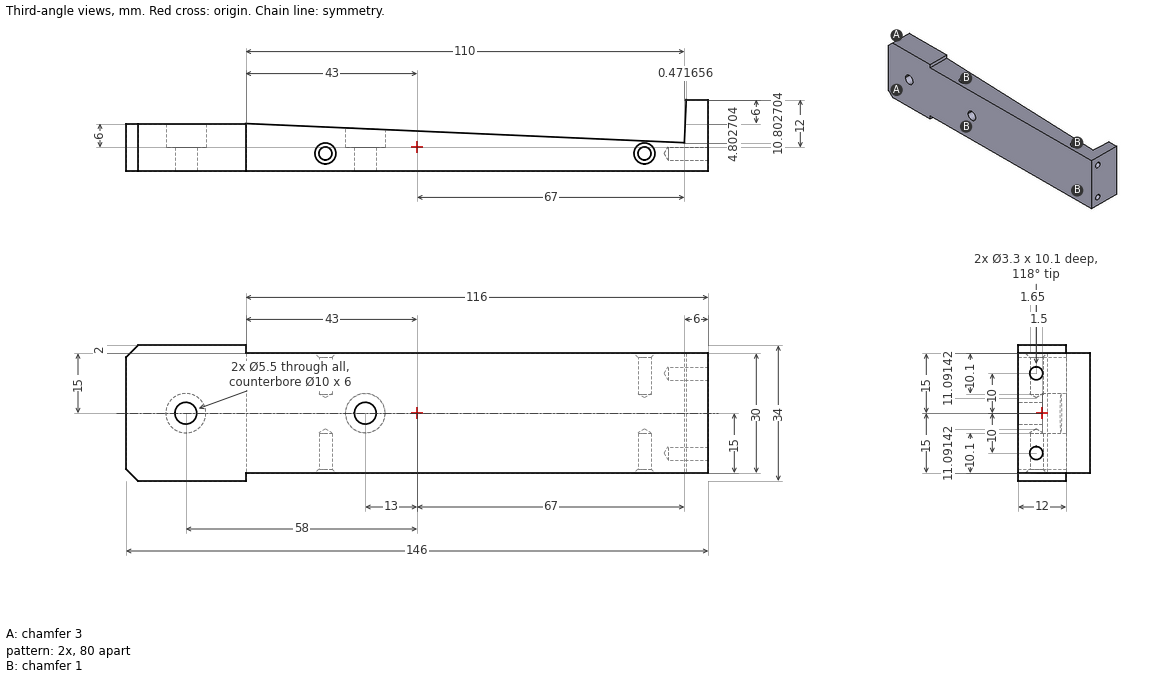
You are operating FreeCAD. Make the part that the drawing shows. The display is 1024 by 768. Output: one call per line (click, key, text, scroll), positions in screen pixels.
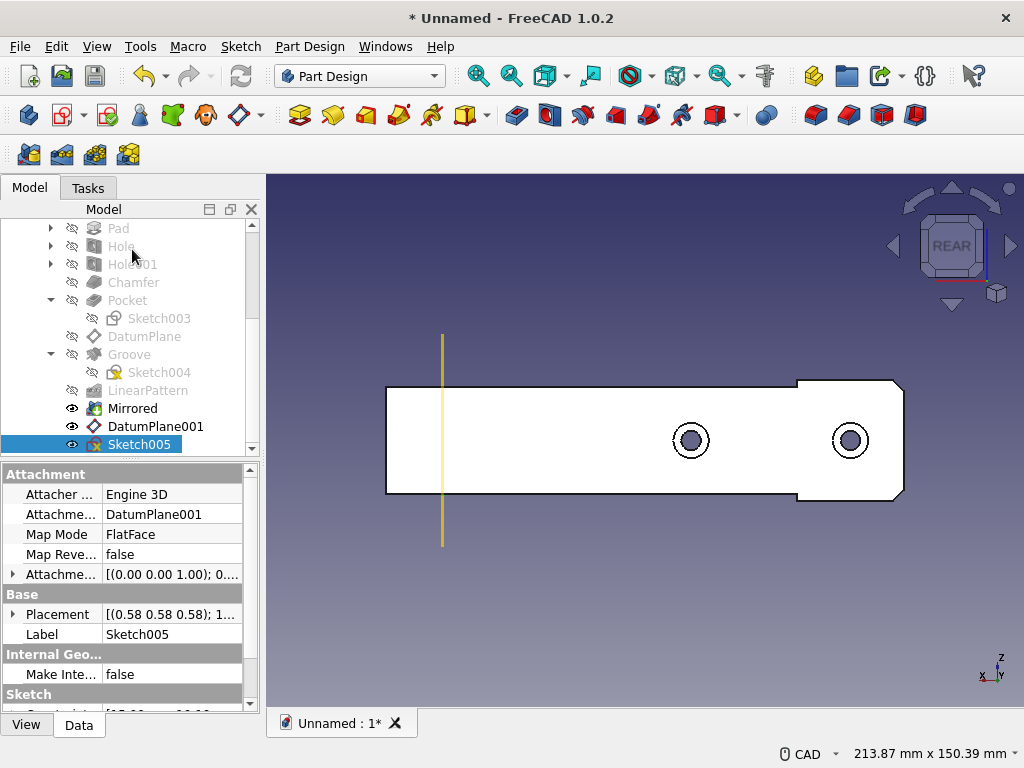
click(583, 116)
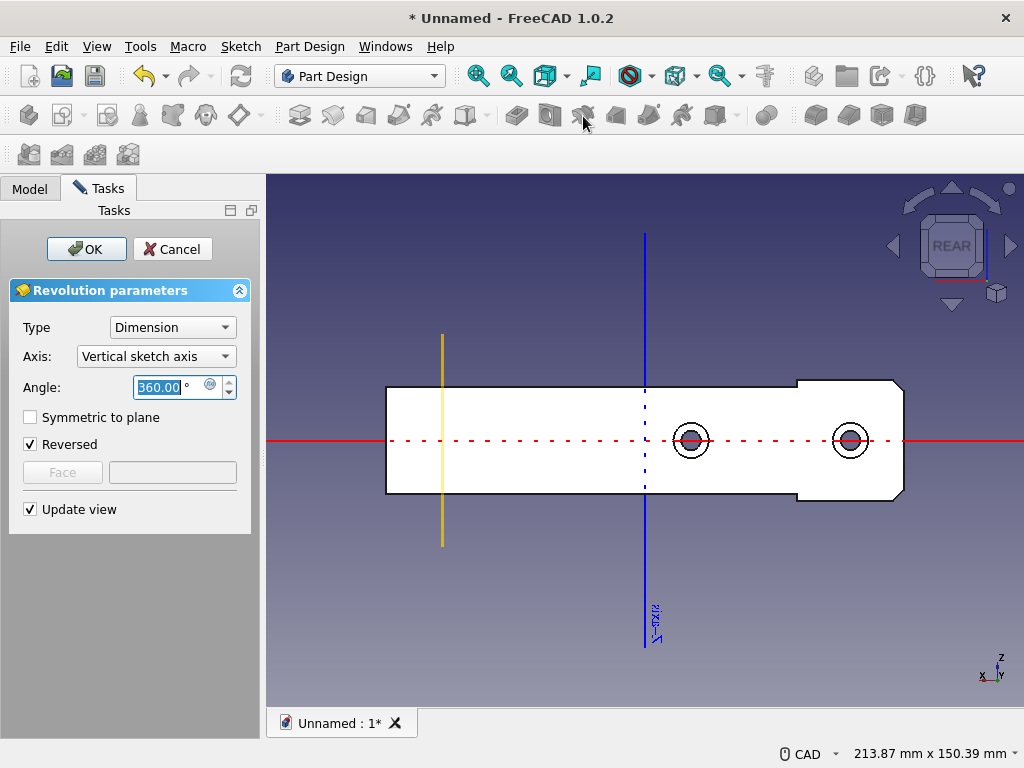
click(157, 356)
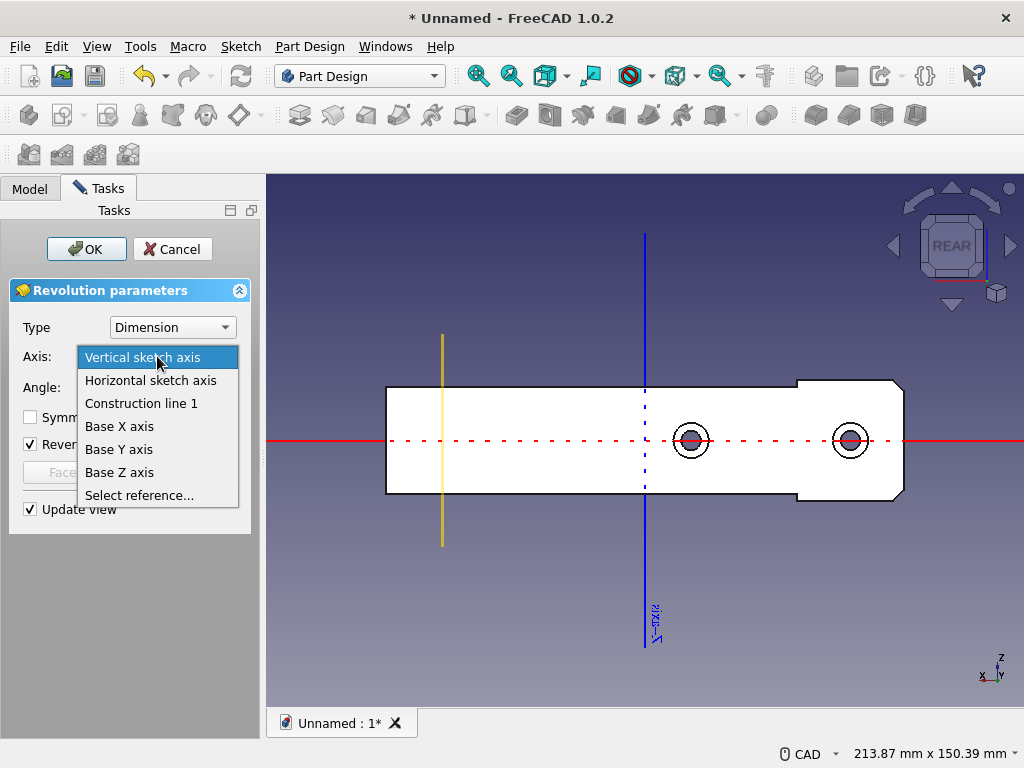
click(156, 404)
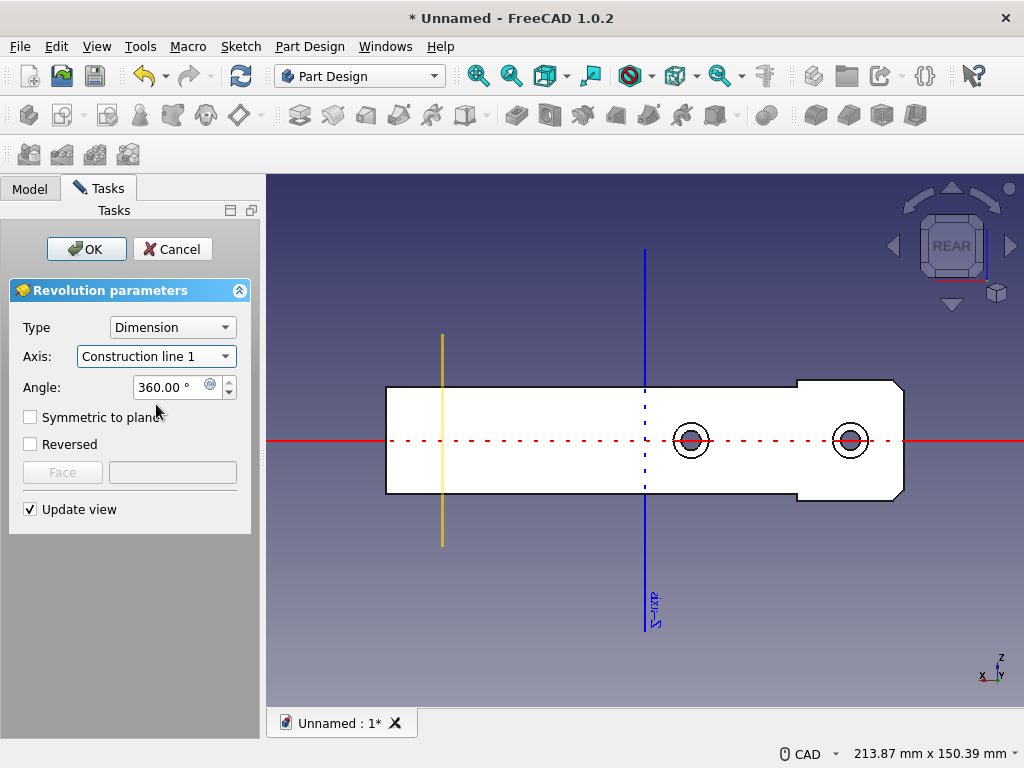
click(87, 249)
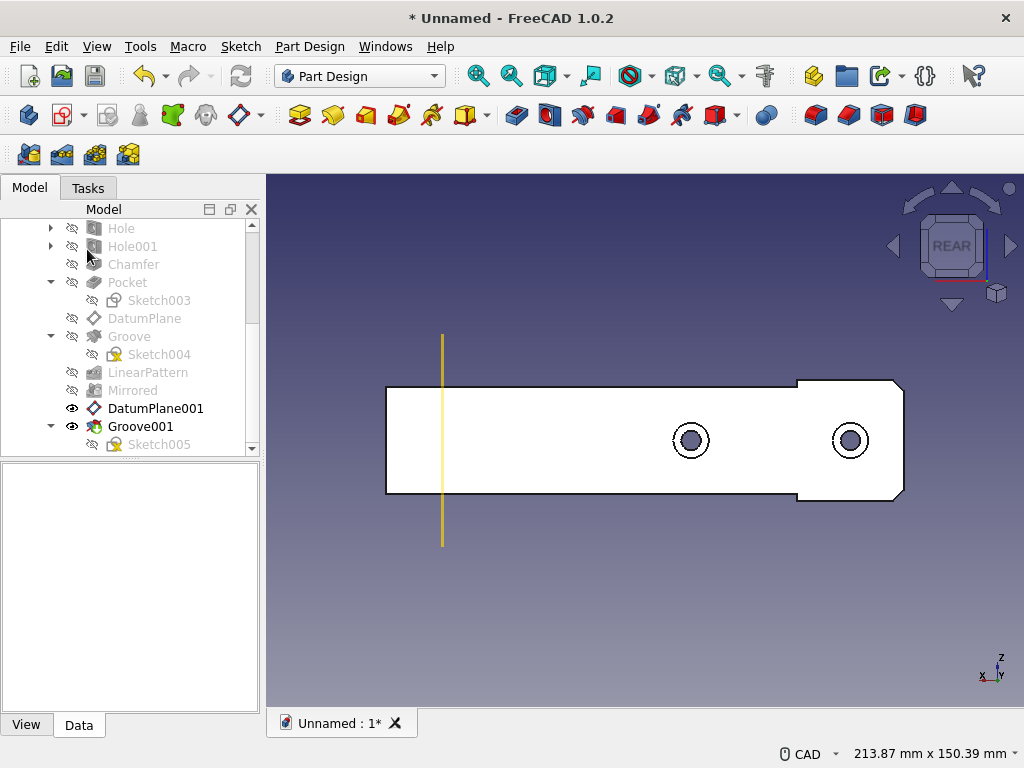
click(117, 408)
key(space)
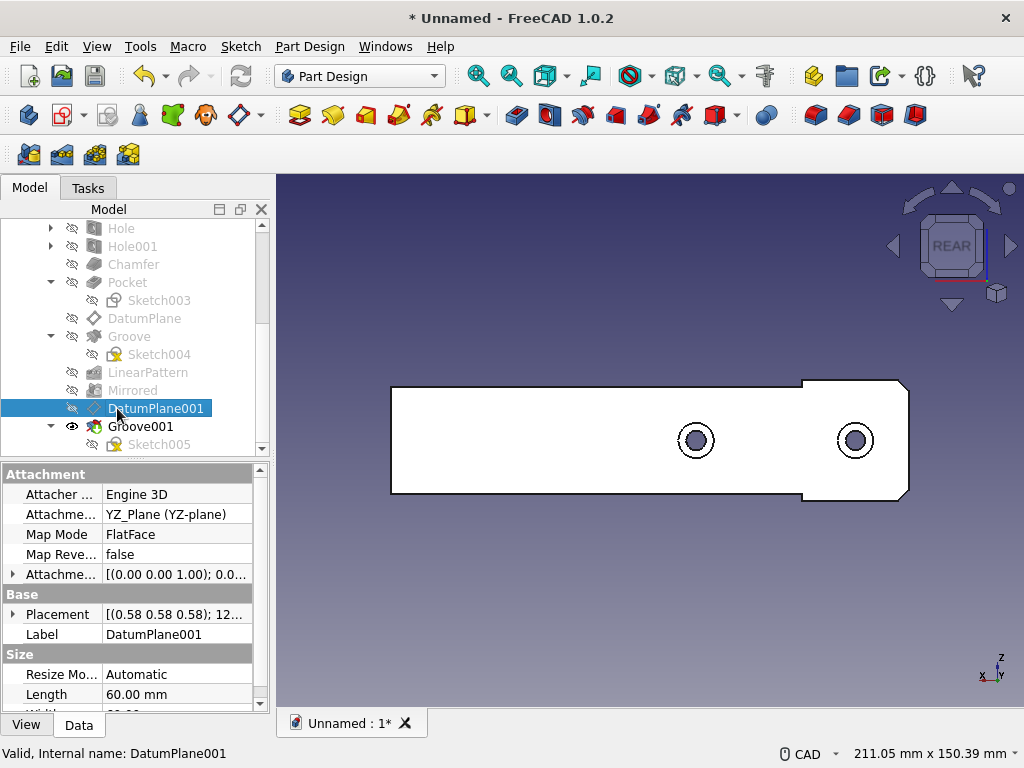
click(502, 439)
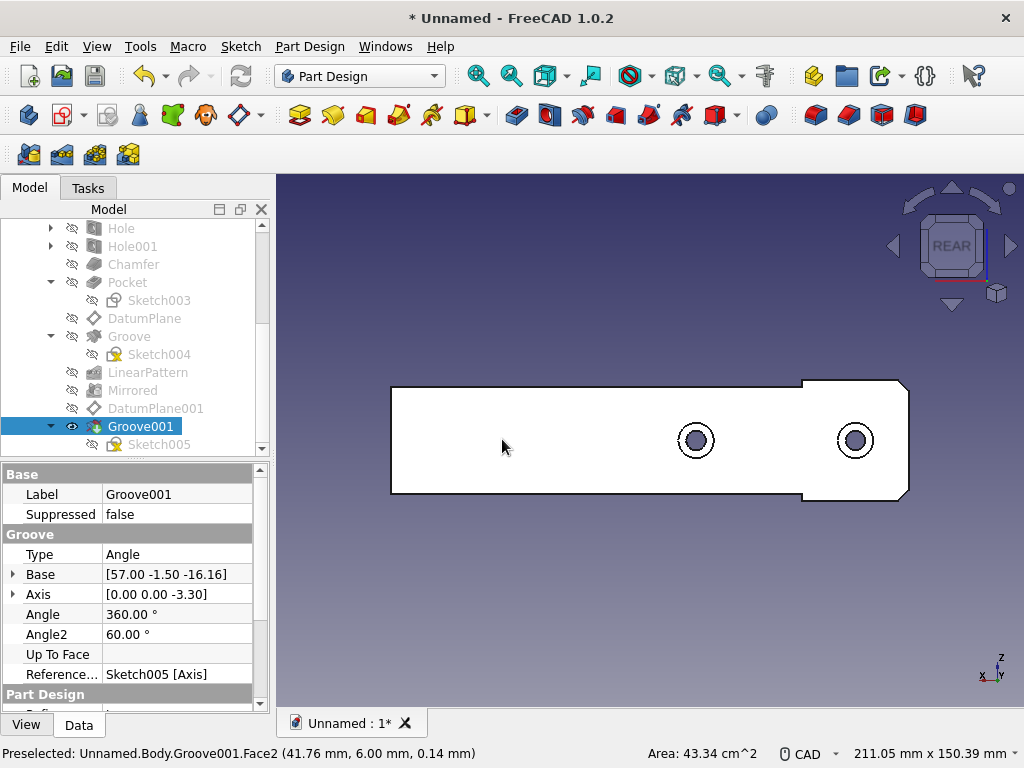
click(62, 116)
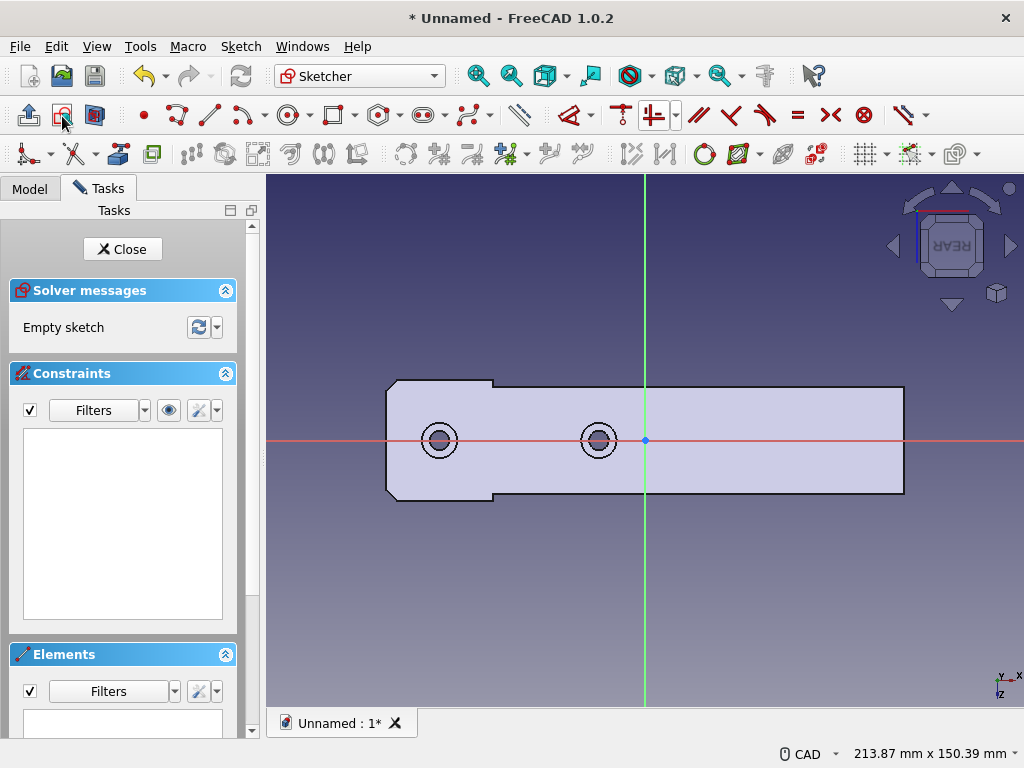
scroll(294, 441, down, 1)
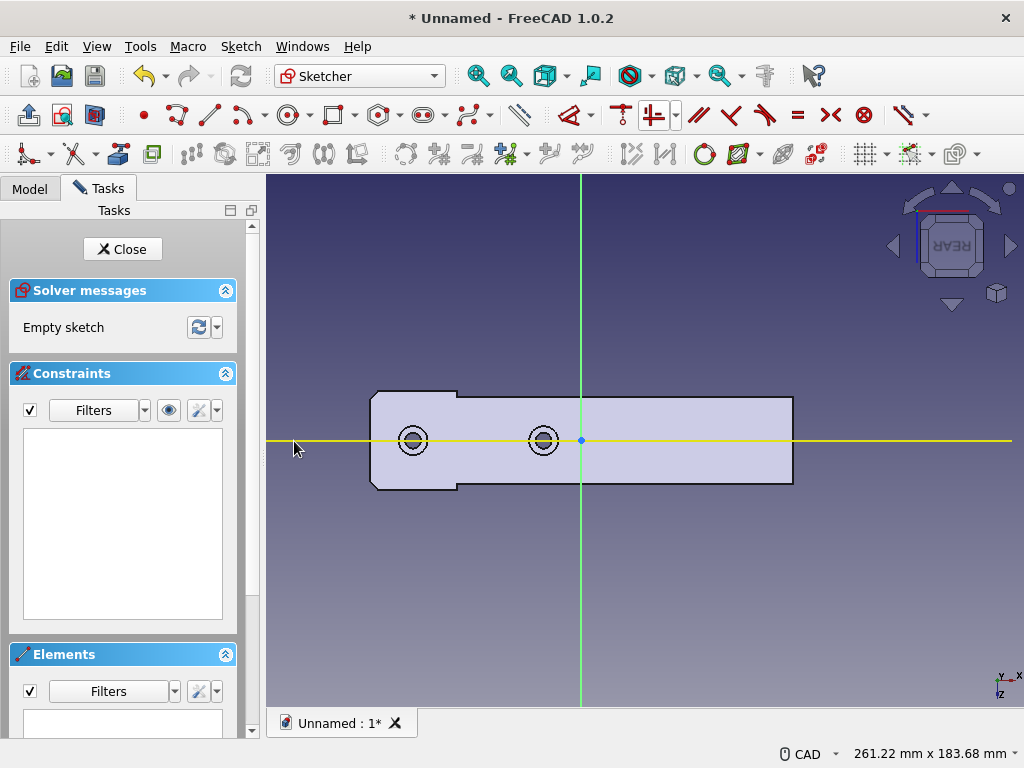
scroll(822, 441, up, 3)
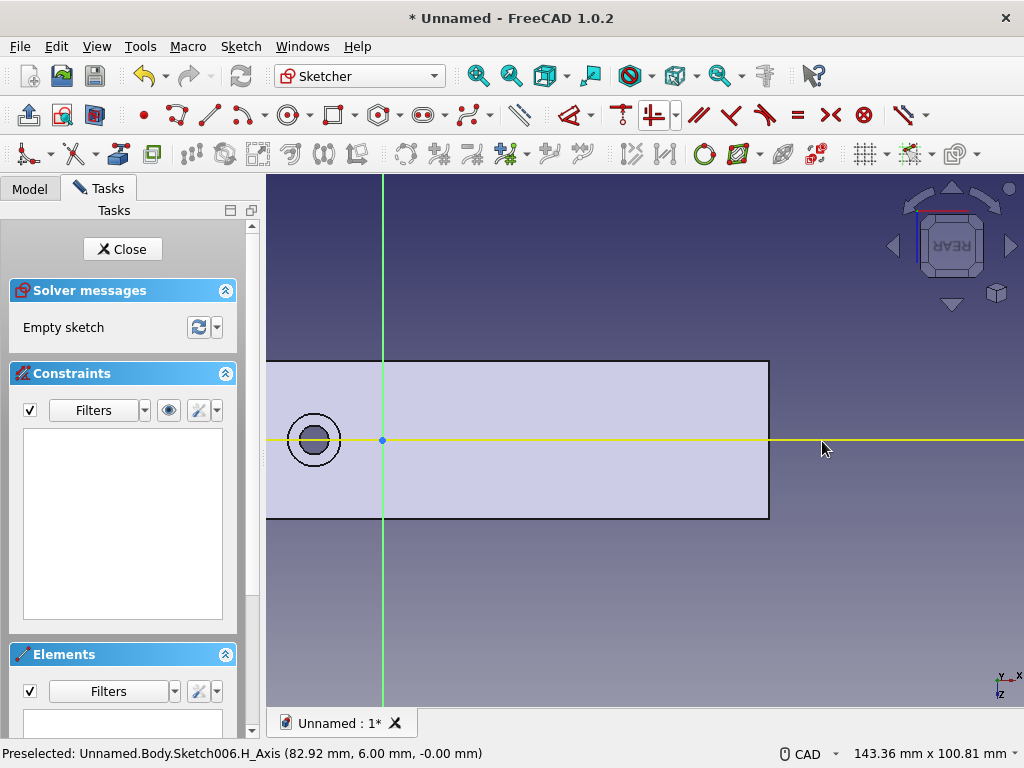
click(332, 116)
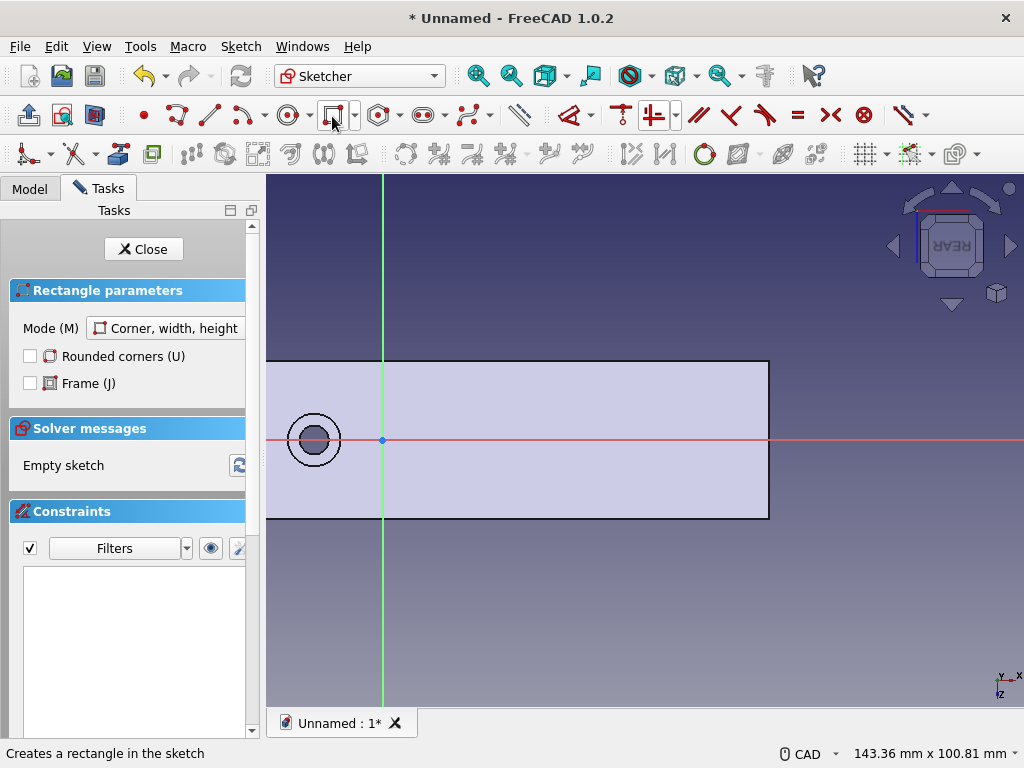
click(737, 361)
move(769, 519)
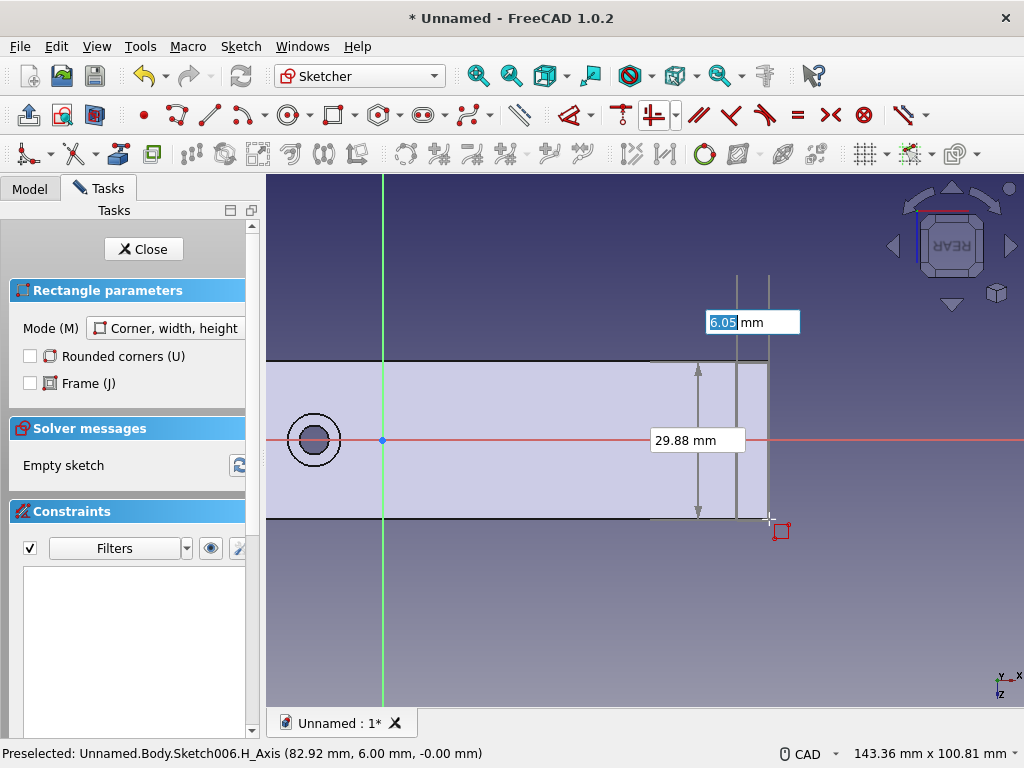
text(6)
key(Tab)
text(30)
key(Return)
key(Escape)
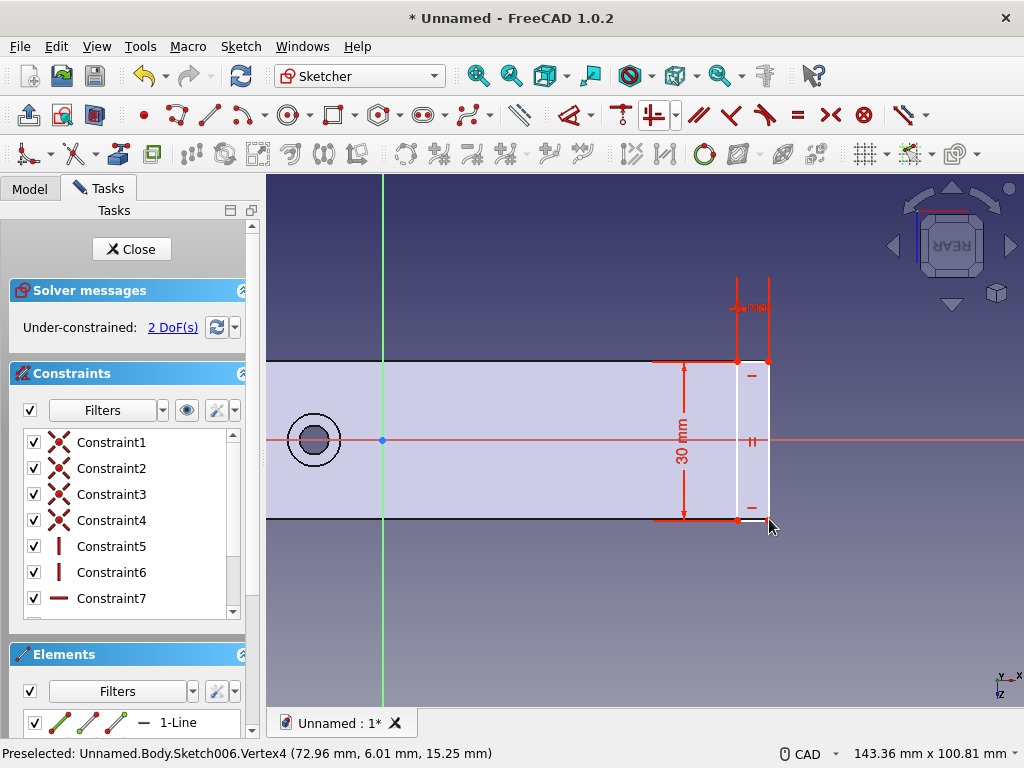
click(568, 116)